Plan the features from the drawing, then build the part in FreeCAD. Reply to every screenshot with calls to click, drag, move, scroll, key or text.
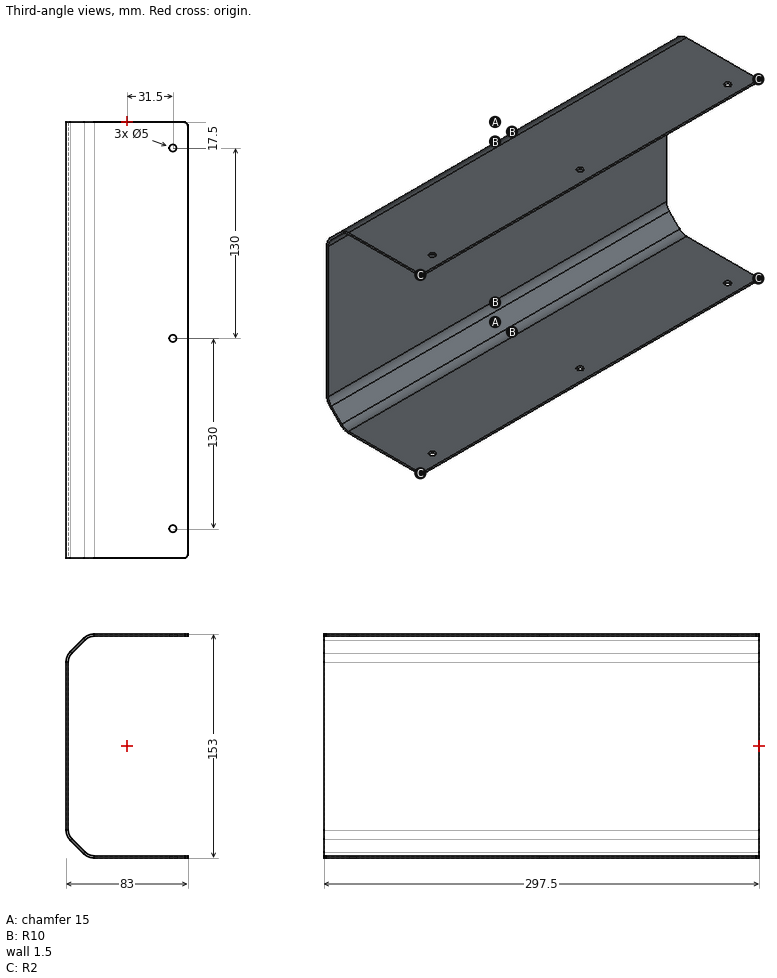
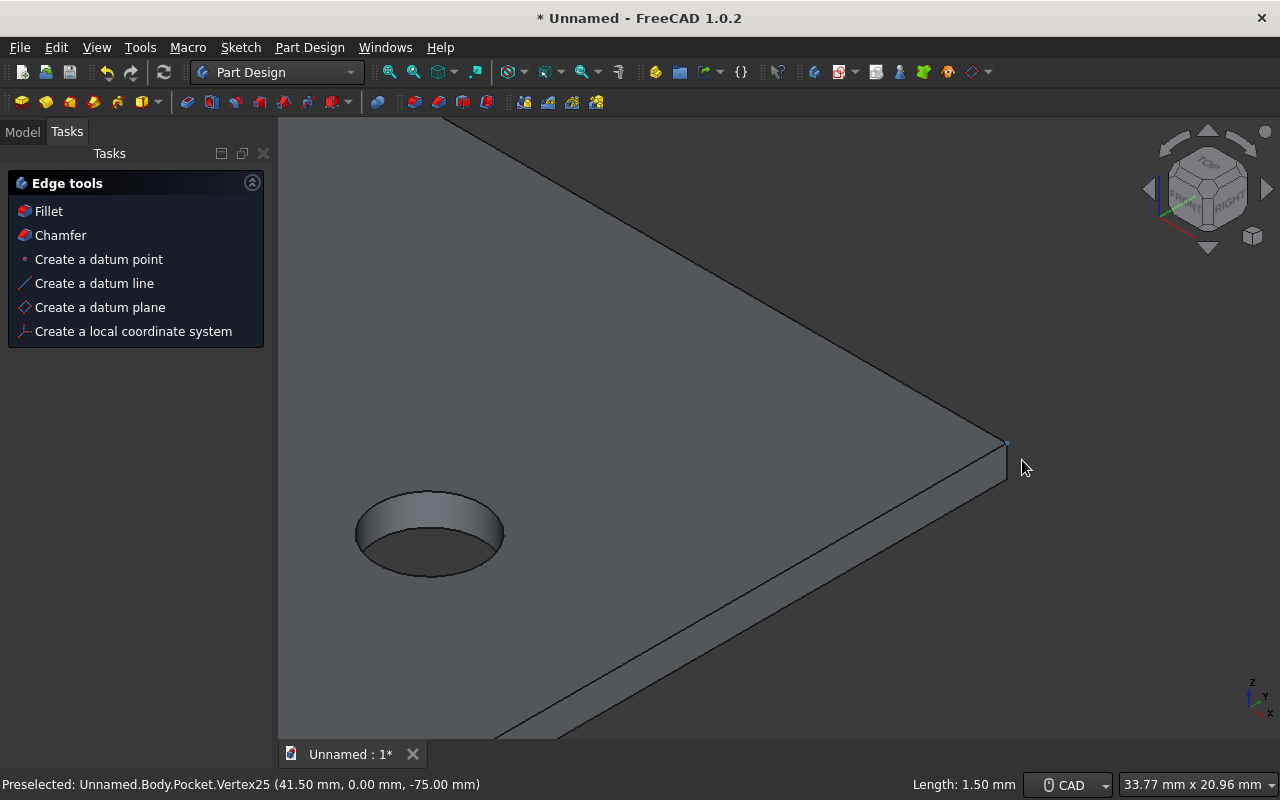
key(v)
key(f)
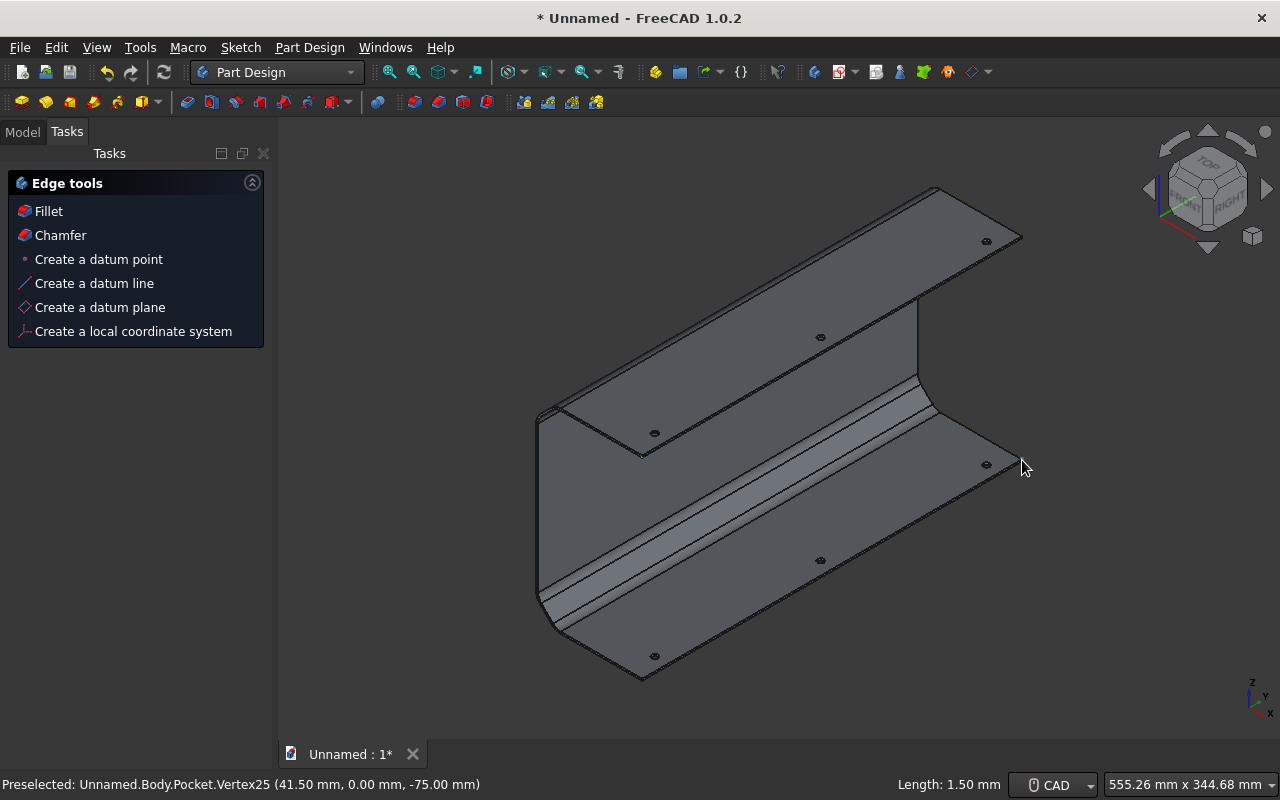
key(1)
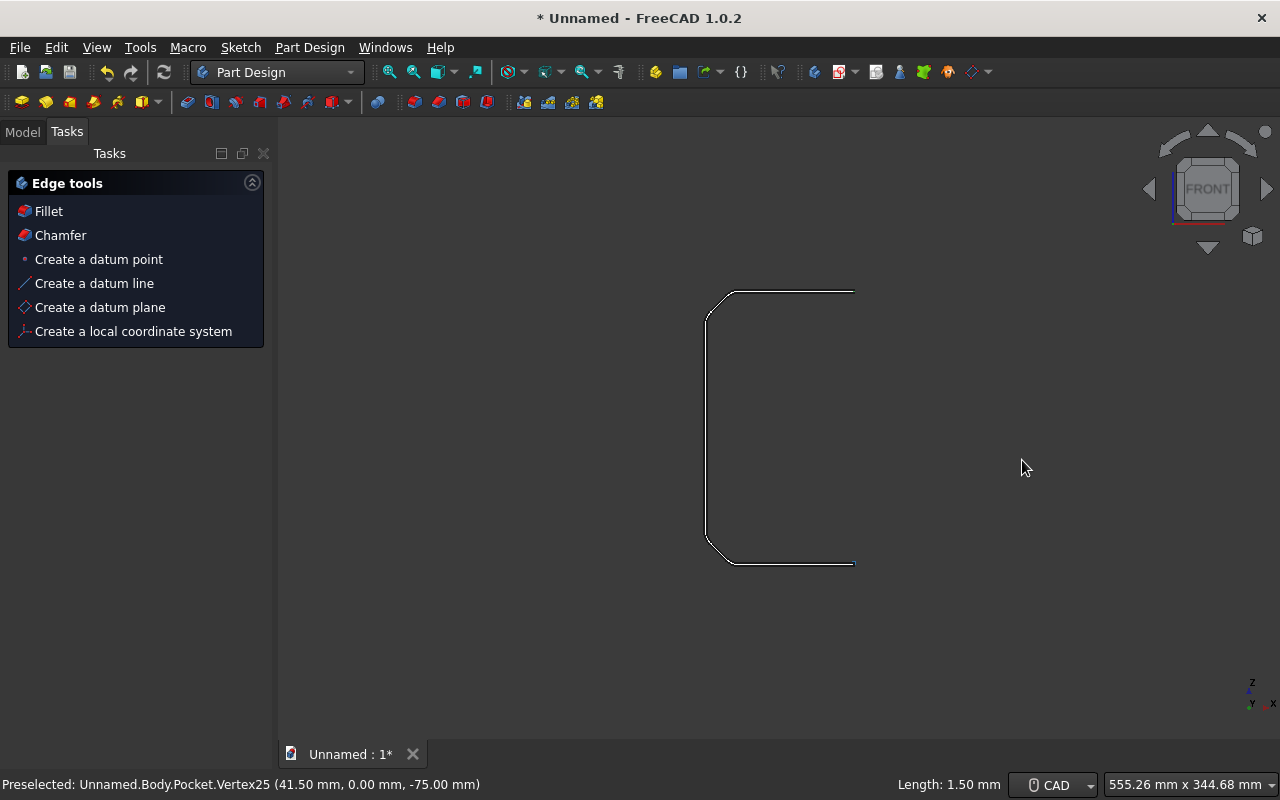
click(390, 72)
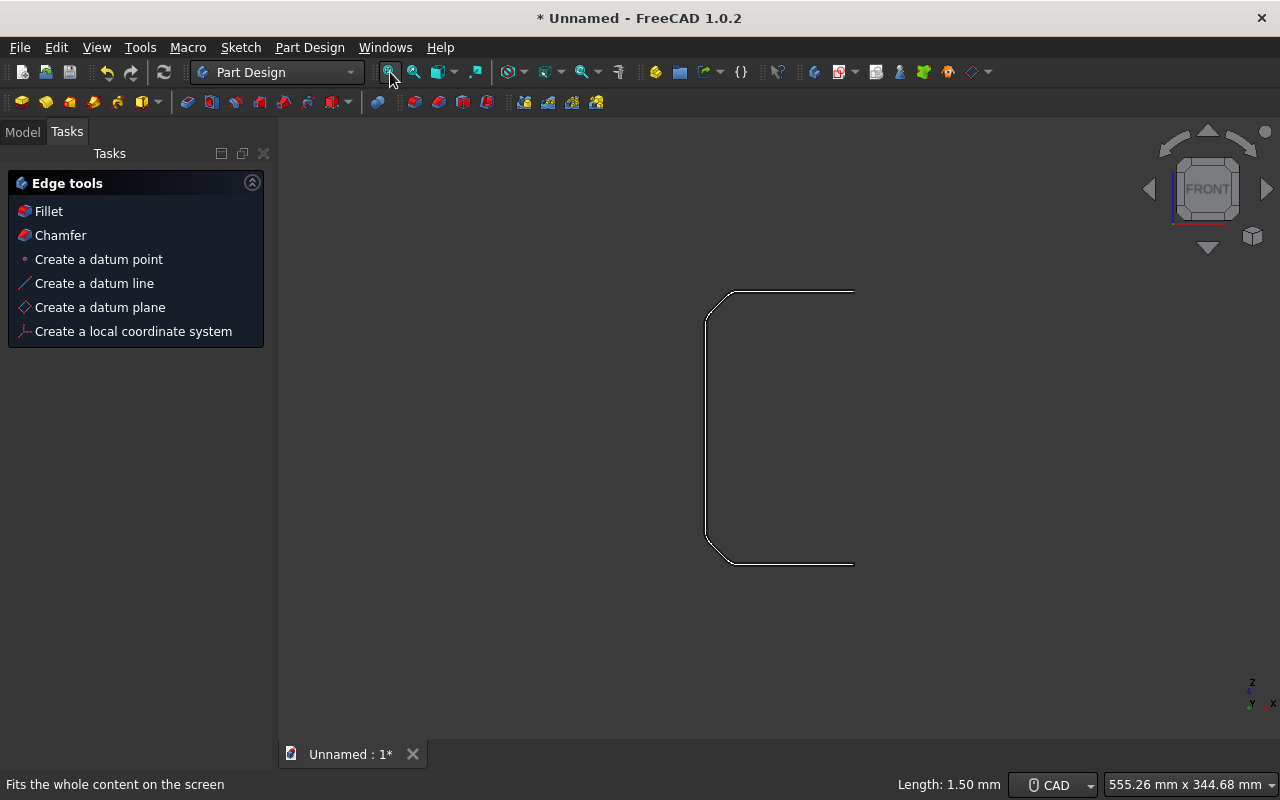
scroll(854, 564, up, 14)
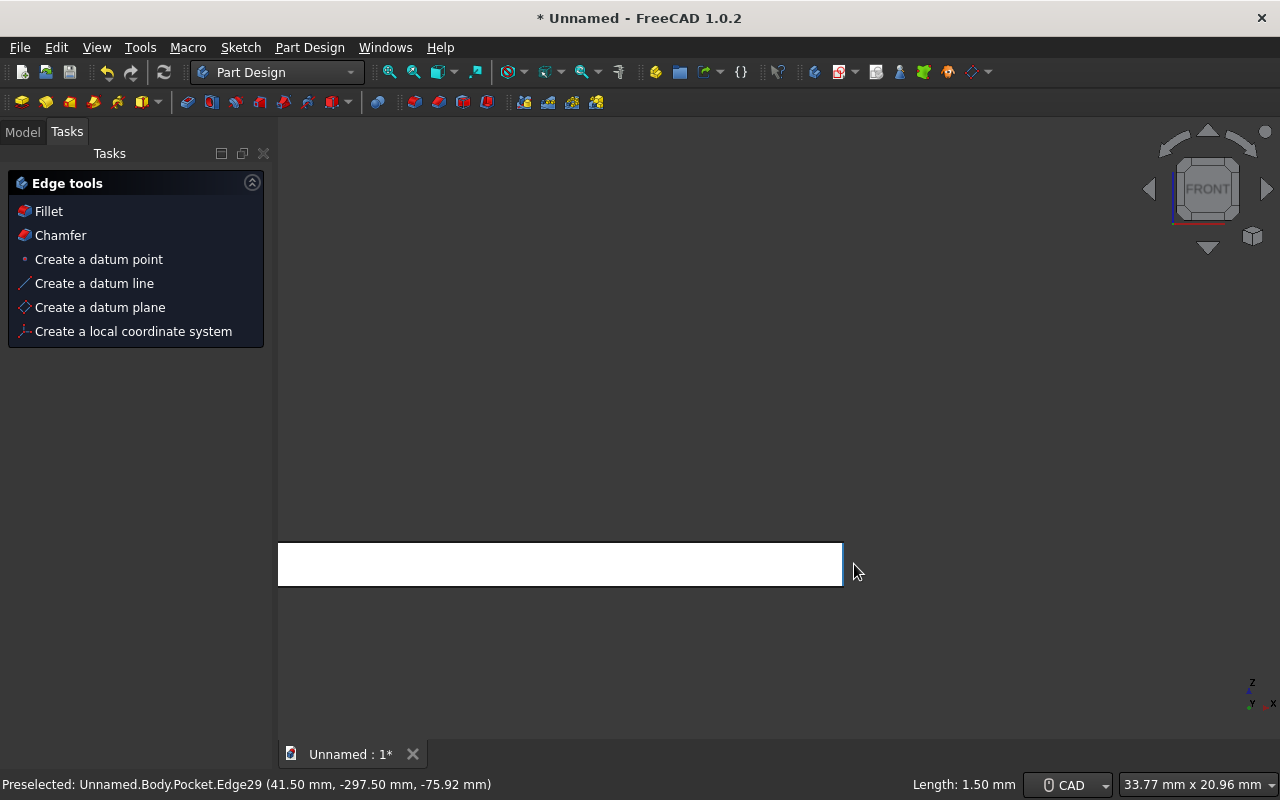
click(843, 563, ctrl)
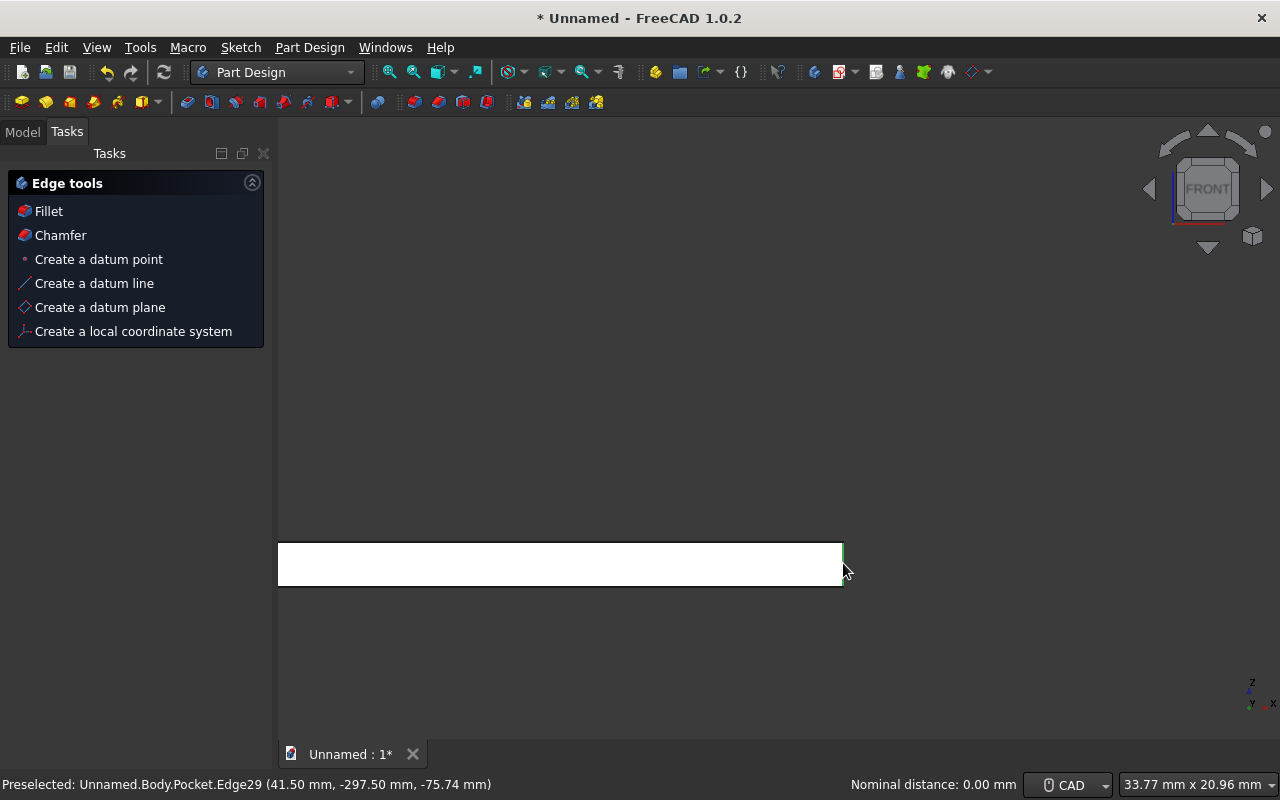
click(390, 72)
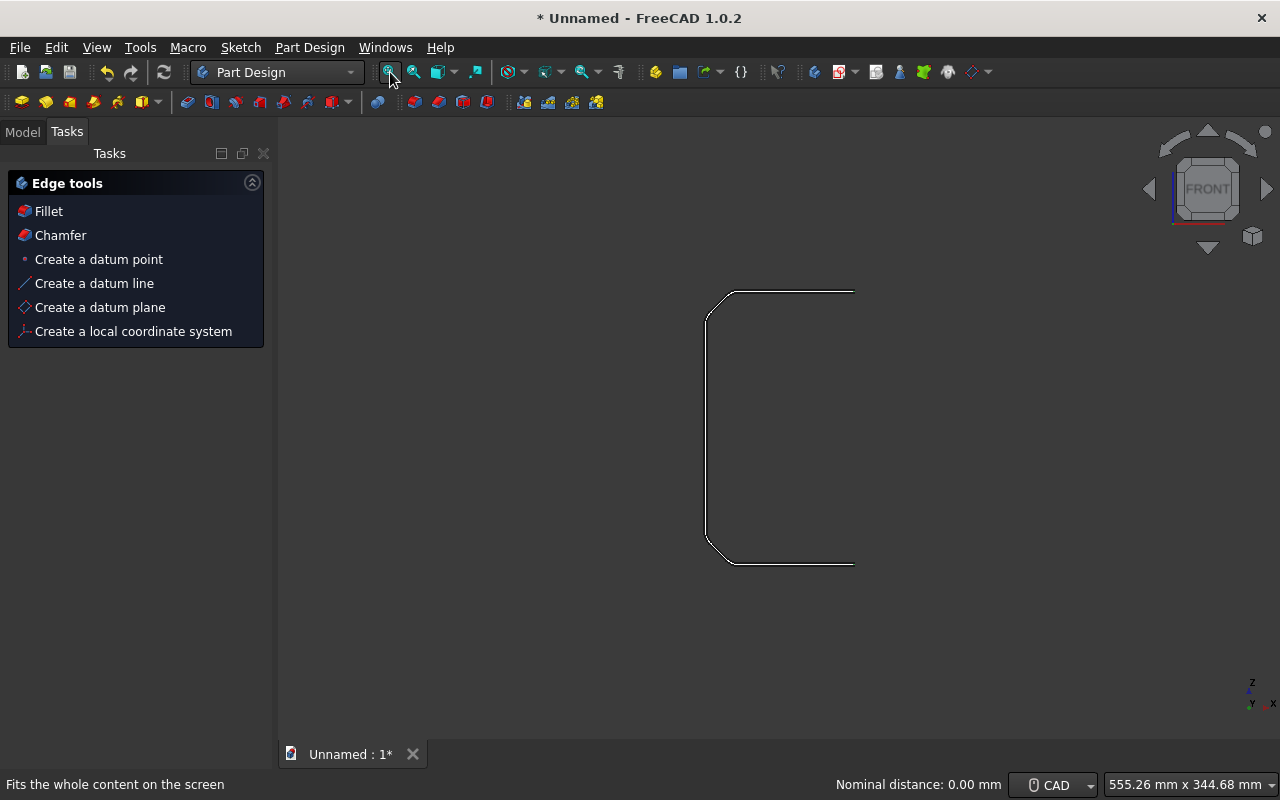
key(3)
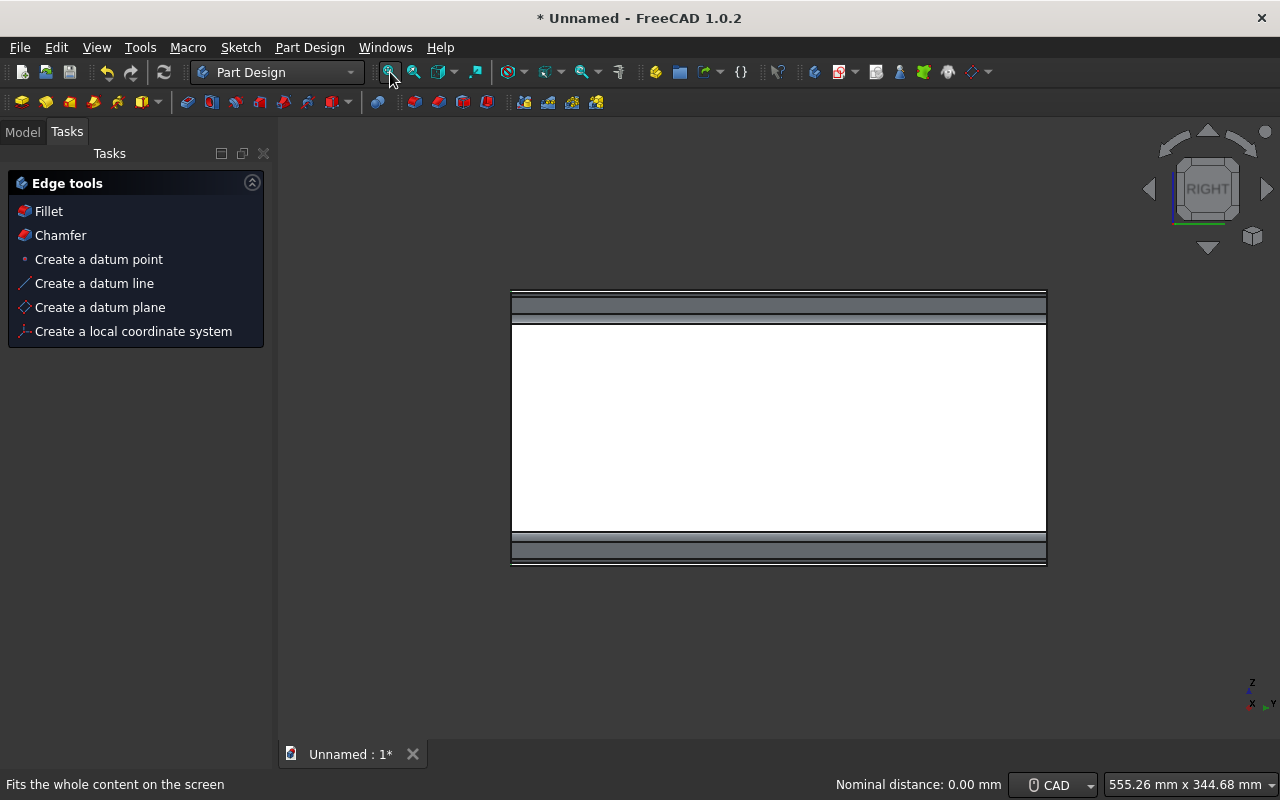
scroll(1047, 564, up, 14)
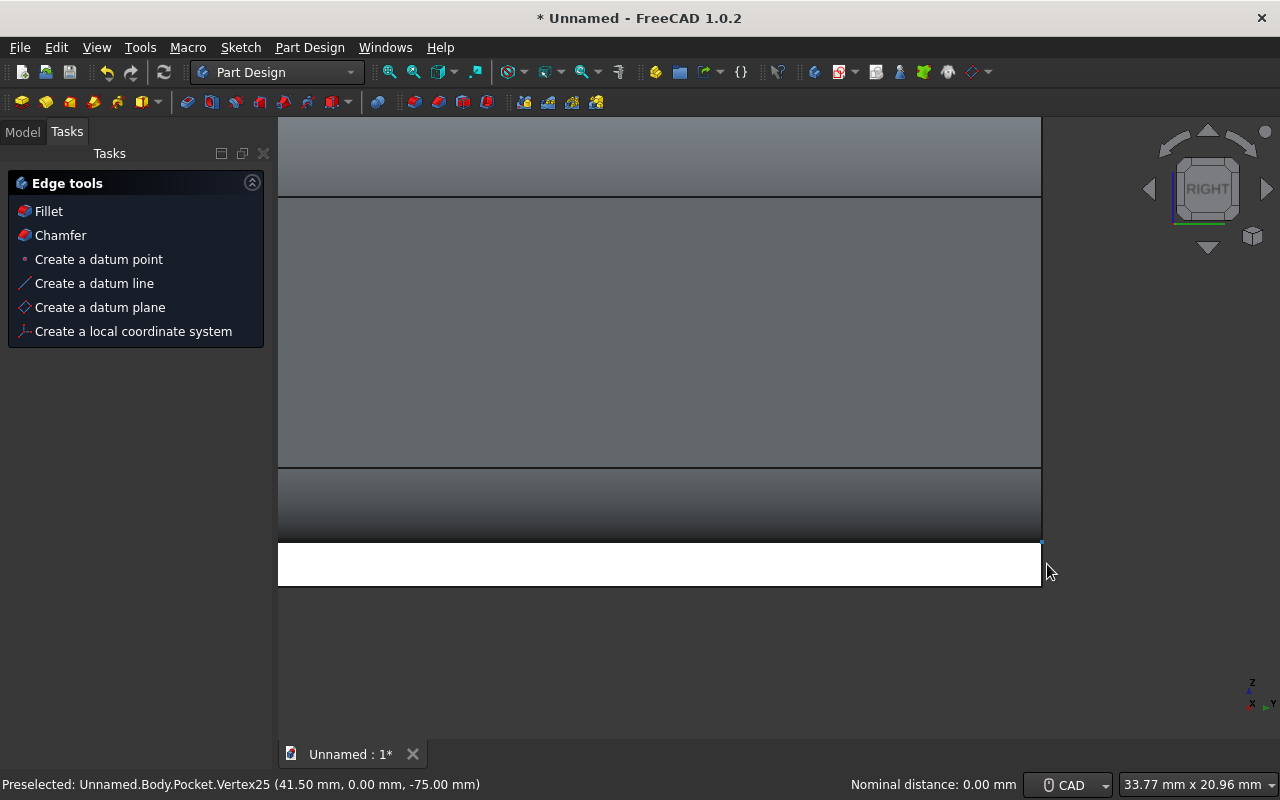
click(1042, 563, ctrl)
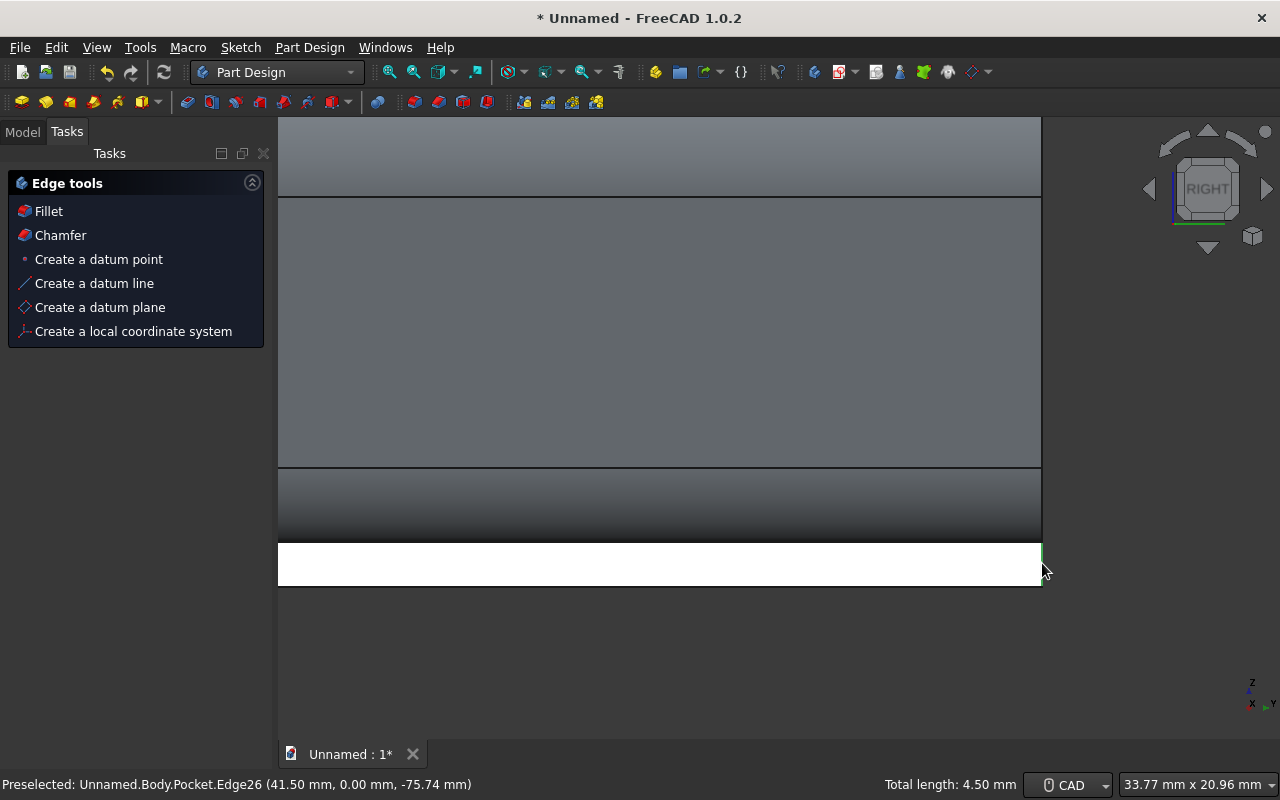
click(390, 72)